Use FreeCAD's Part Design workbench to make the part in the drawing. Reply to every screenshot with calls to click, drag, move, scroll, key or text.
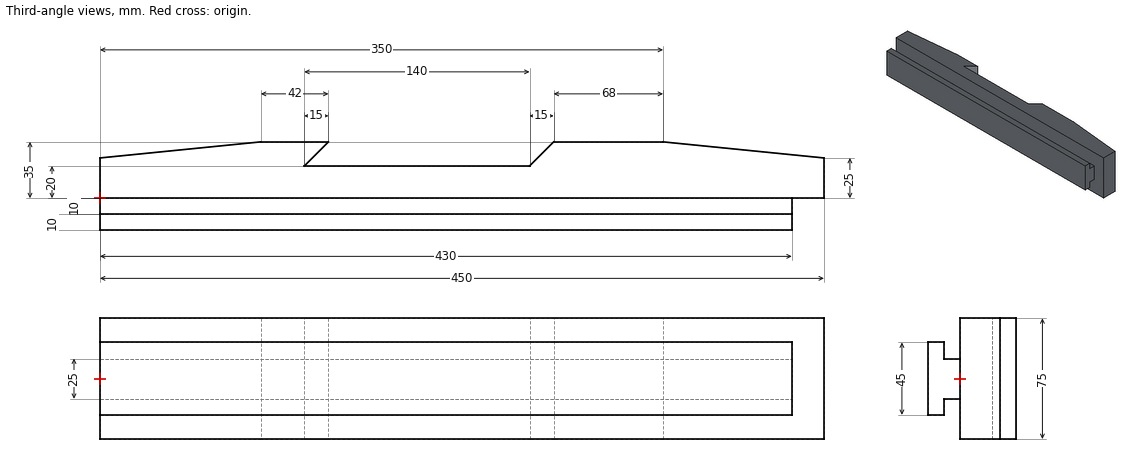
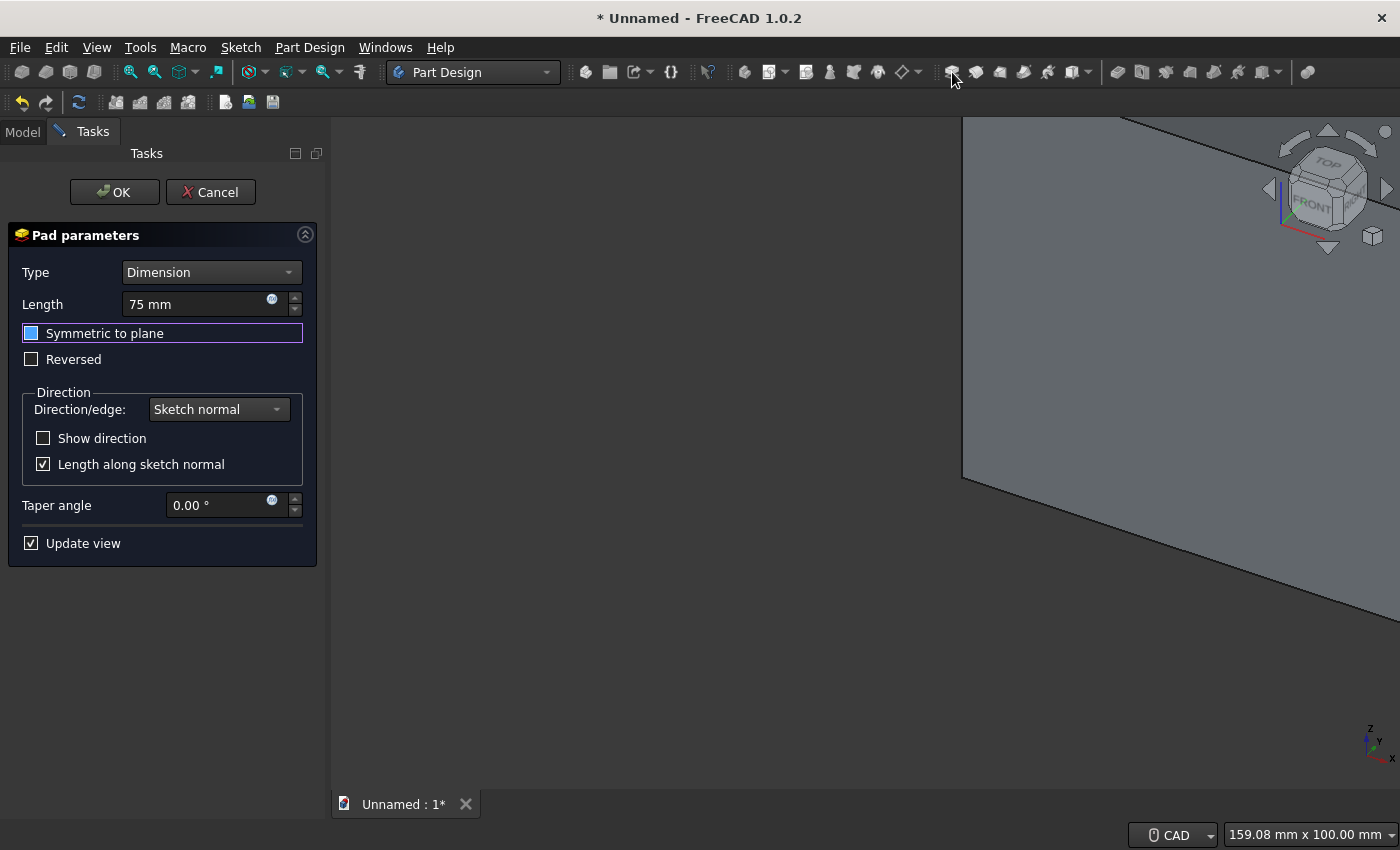
click(30, 333)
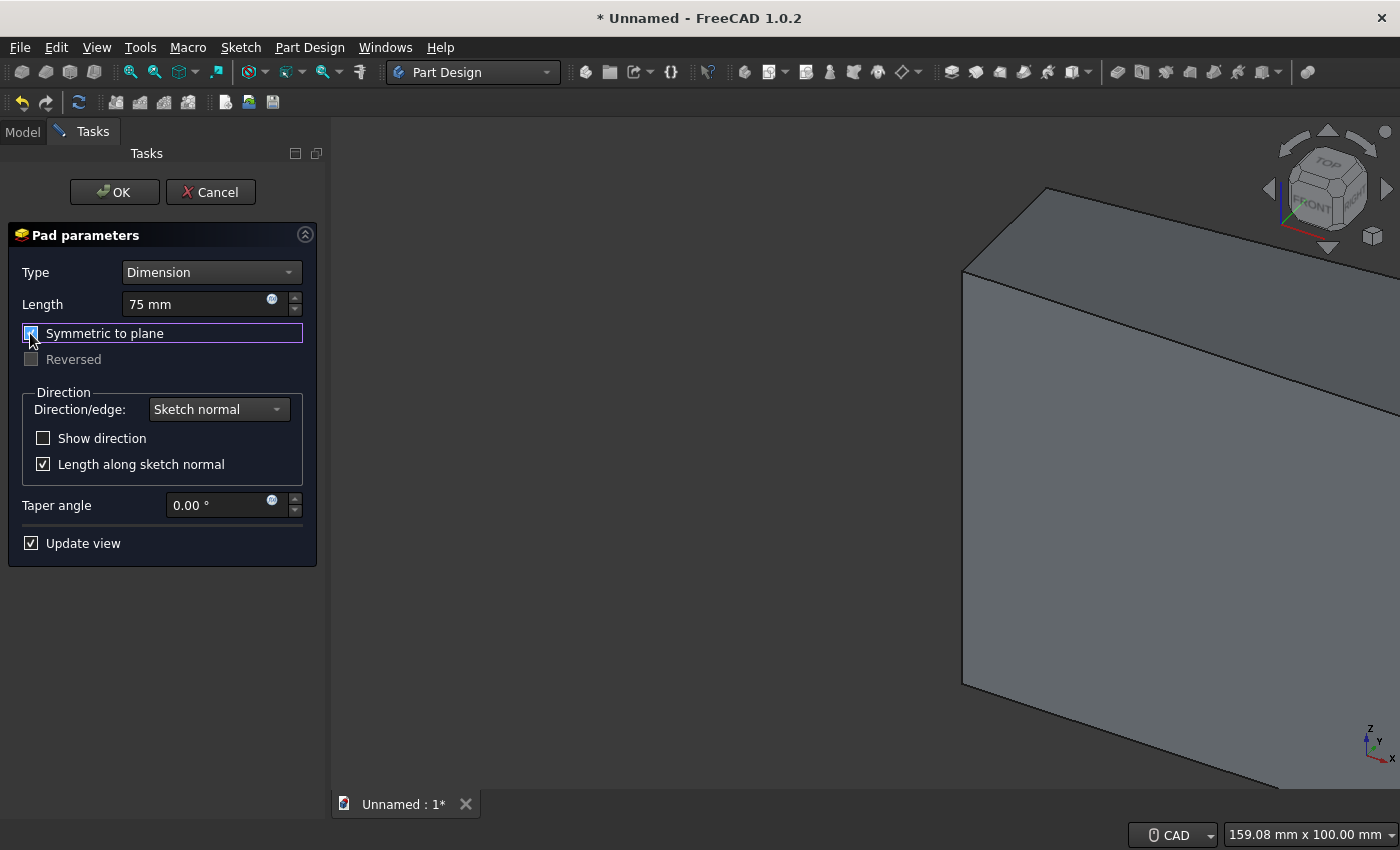
click(115, 192)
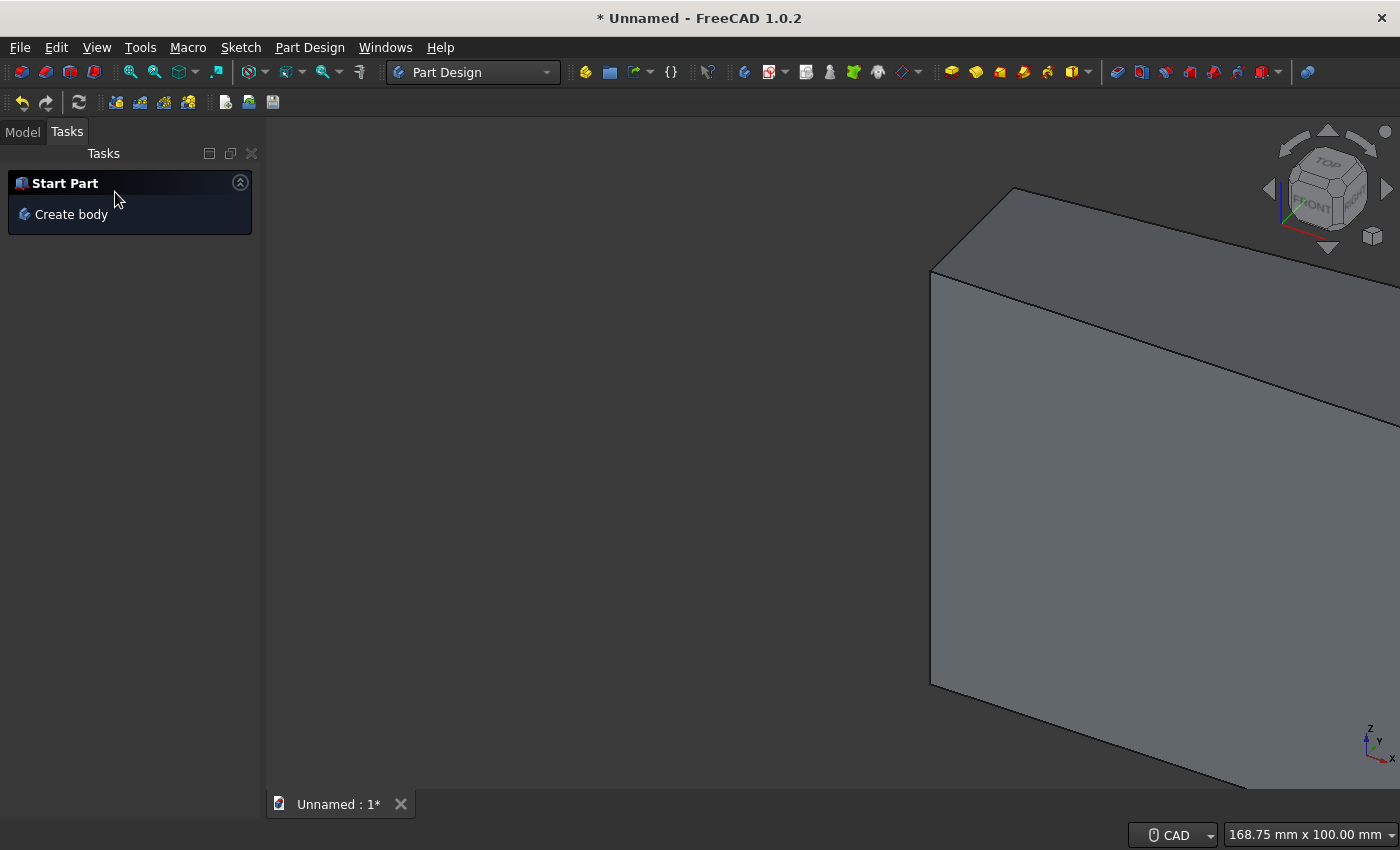
click(132, 72)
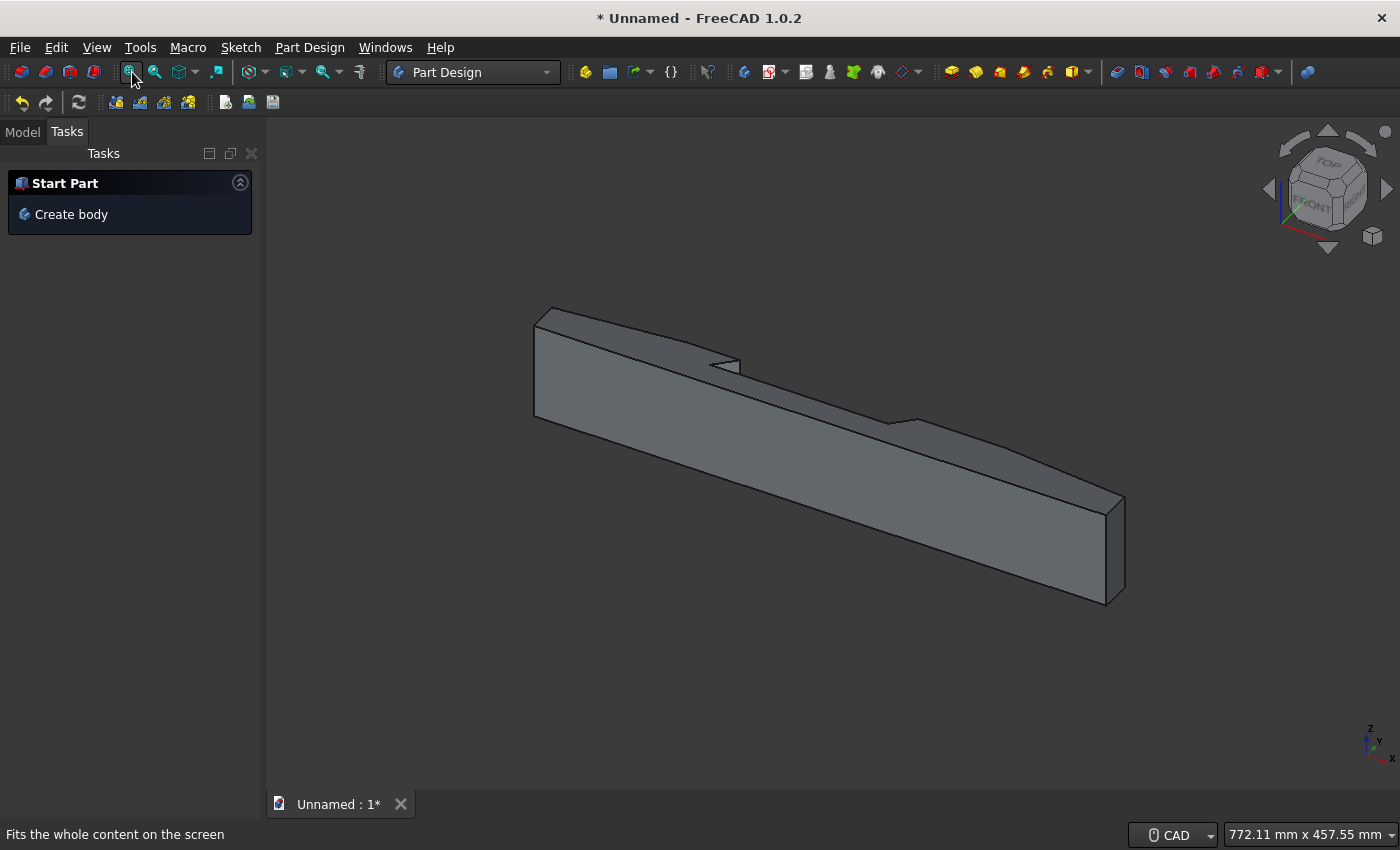
click(770, 72)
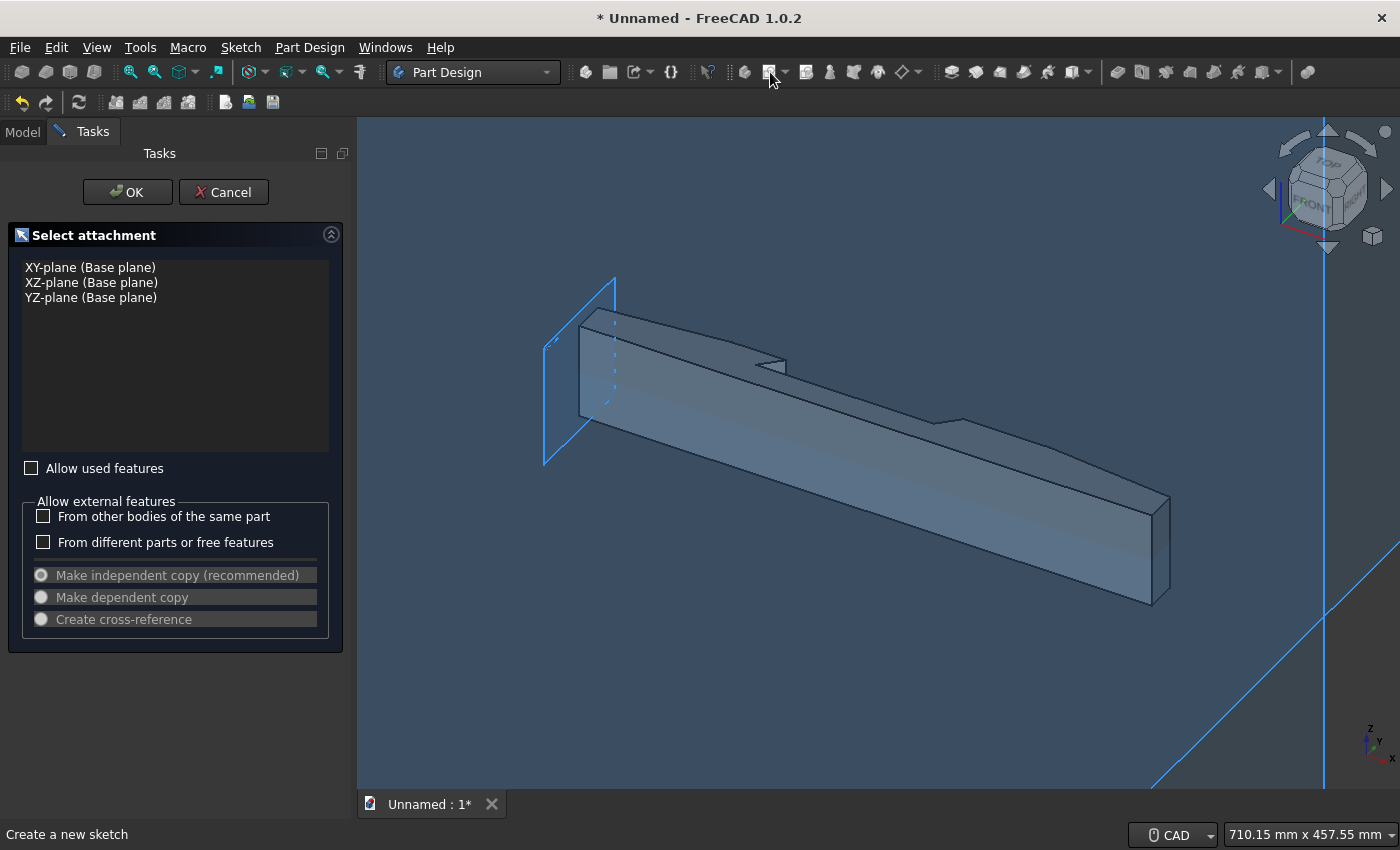
click(82, 268)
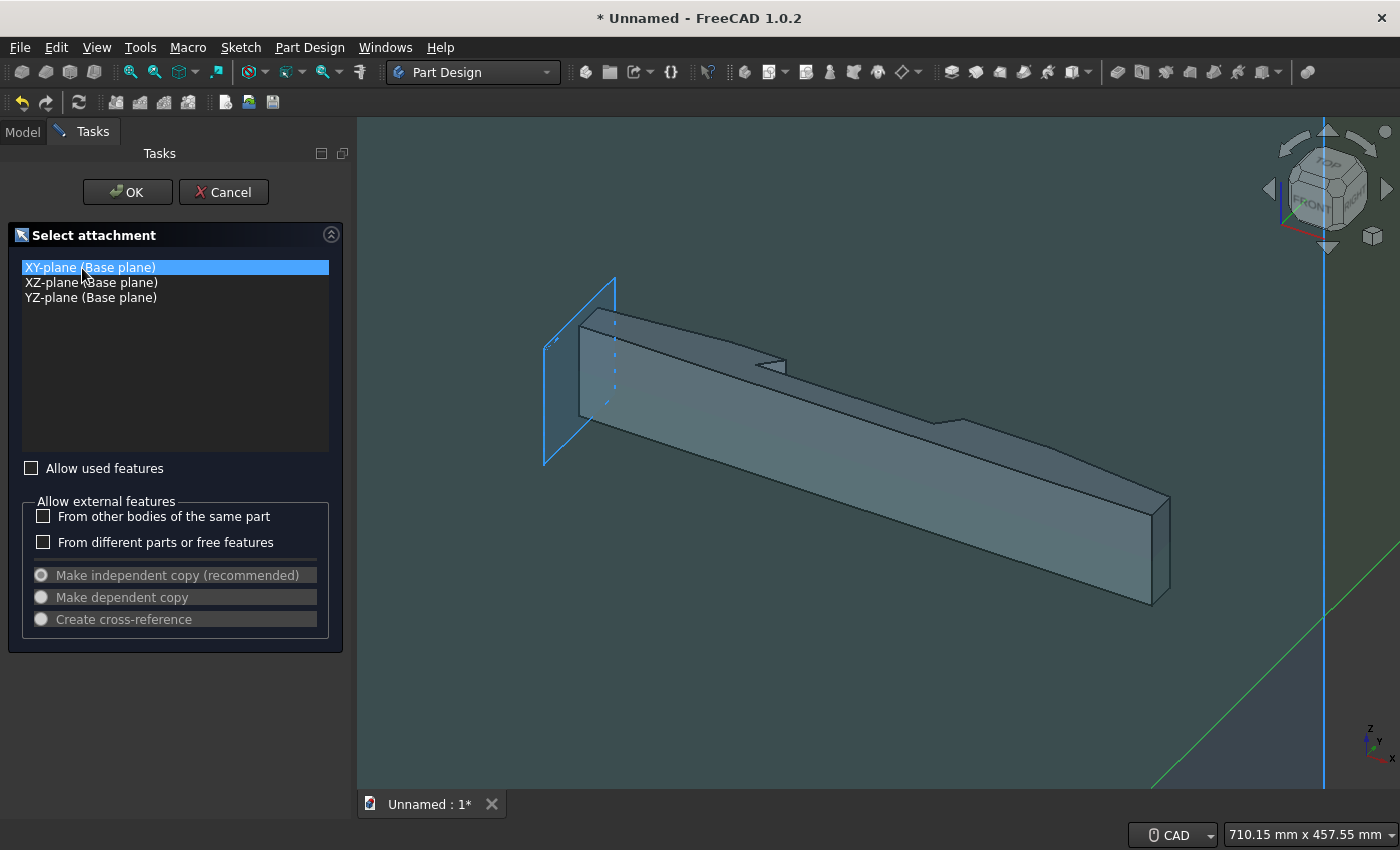
click(128, 192)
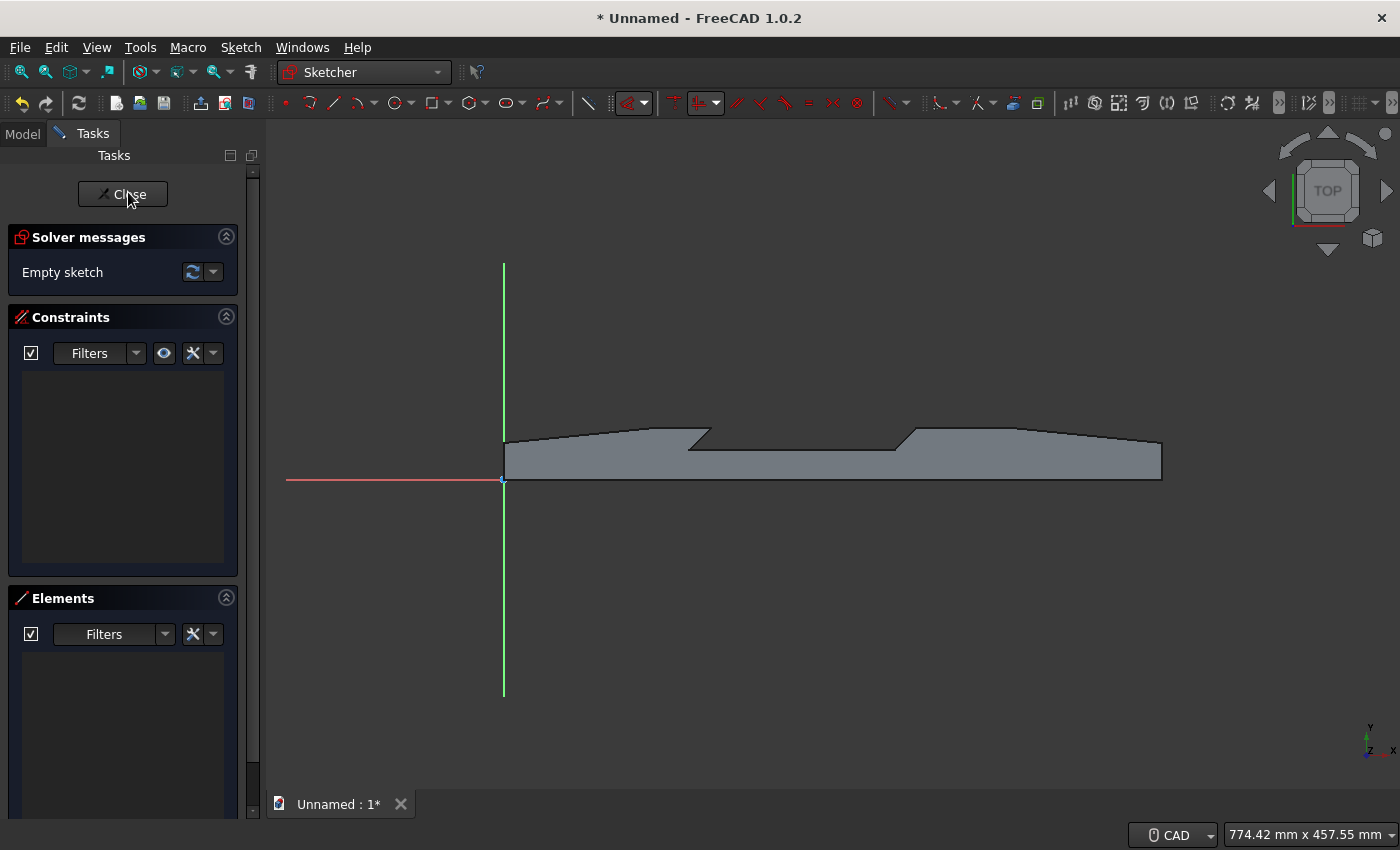
click(250, 104)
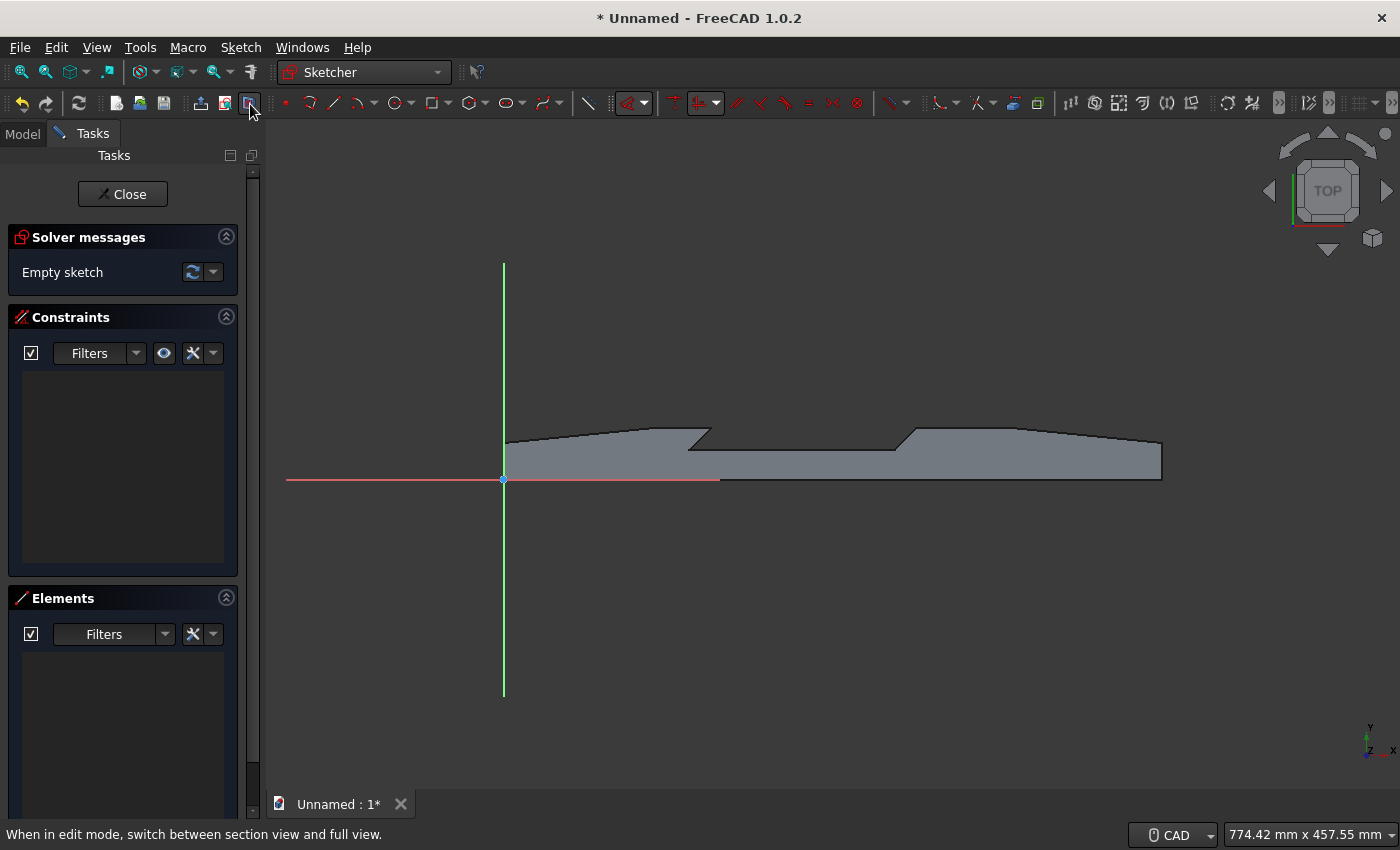
click(432, 104)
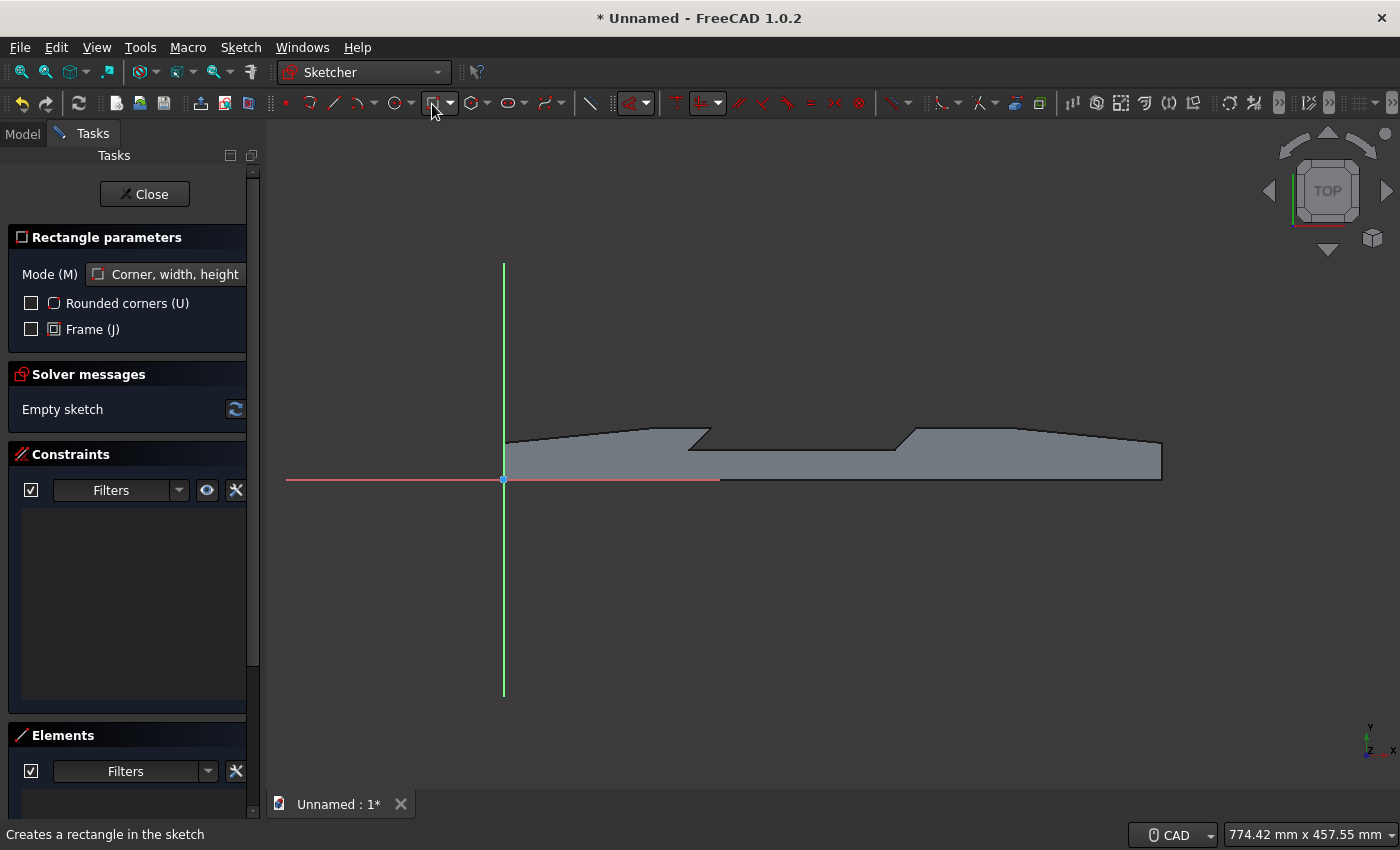
click(504, 480)
click(1133, 494)
key(Escape)